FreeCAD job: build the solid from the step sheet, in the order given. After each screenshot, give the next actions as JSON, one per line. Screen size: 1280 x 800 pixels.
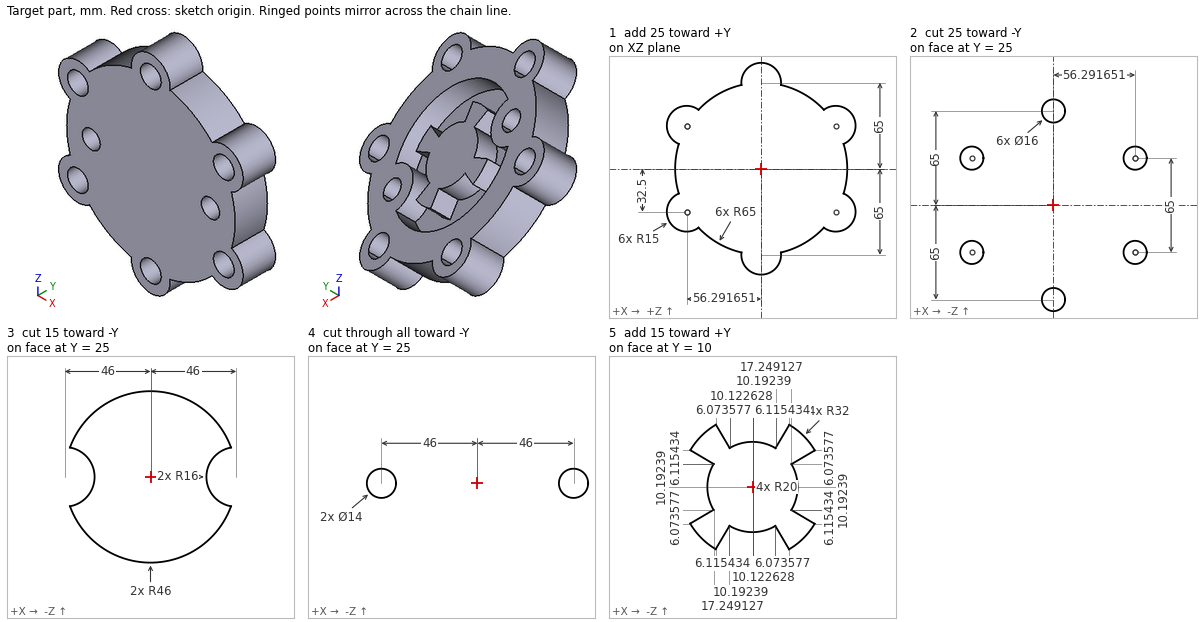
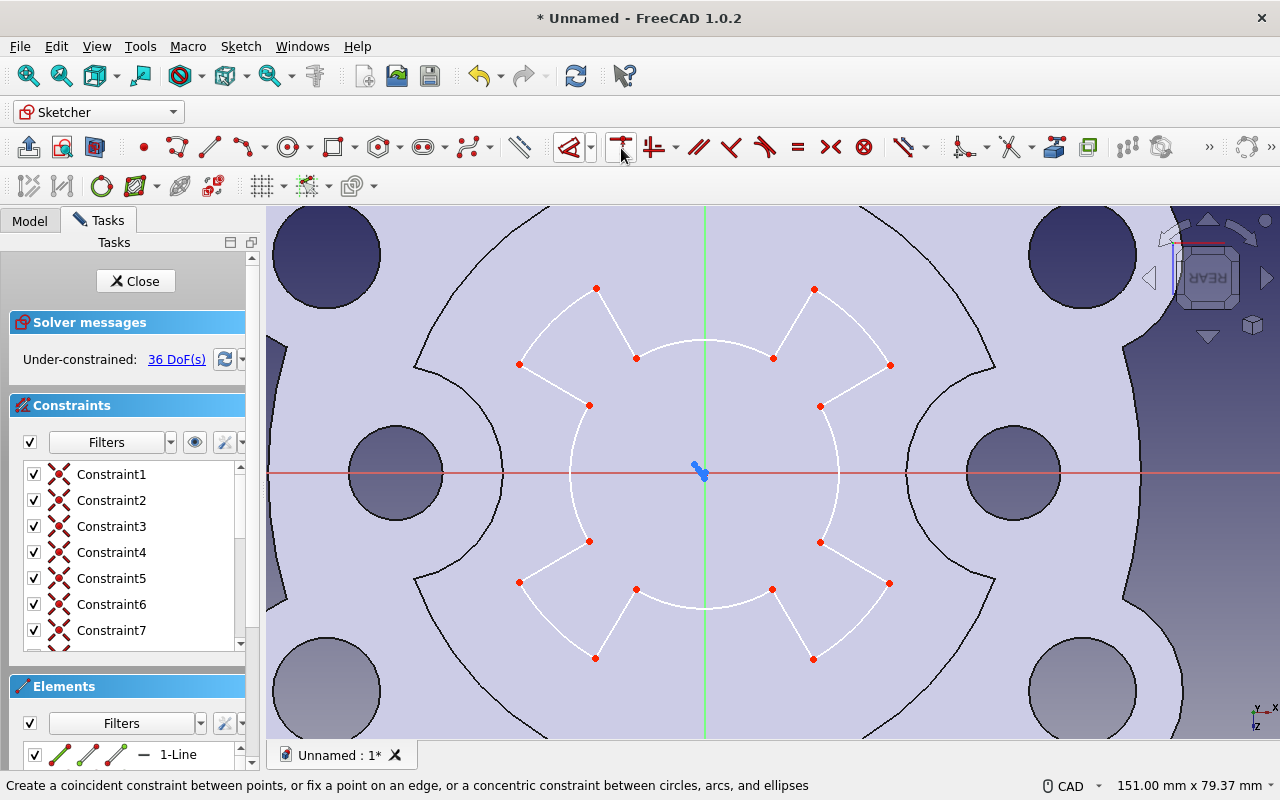
{"action": "left_click", "coordinate": [836, 503]}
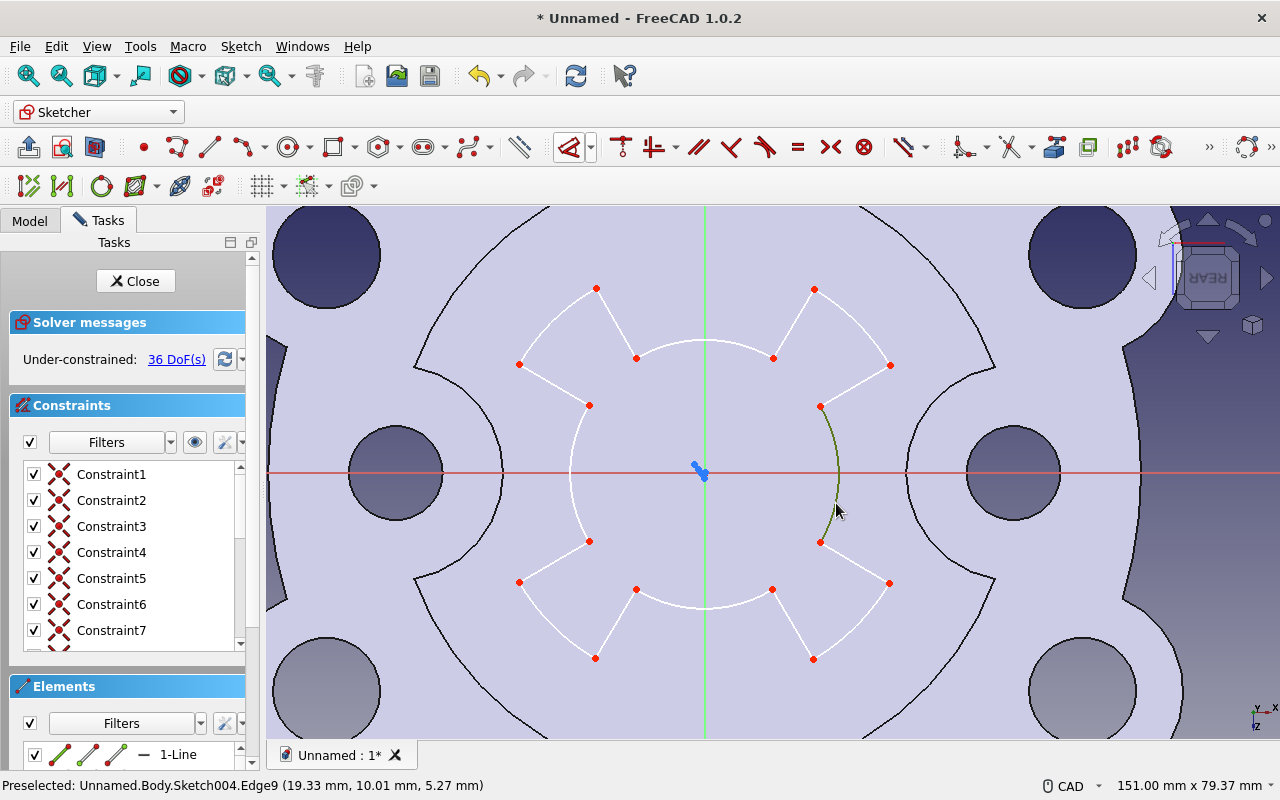
{"action": "left_click", "coordinate": [569, 307]}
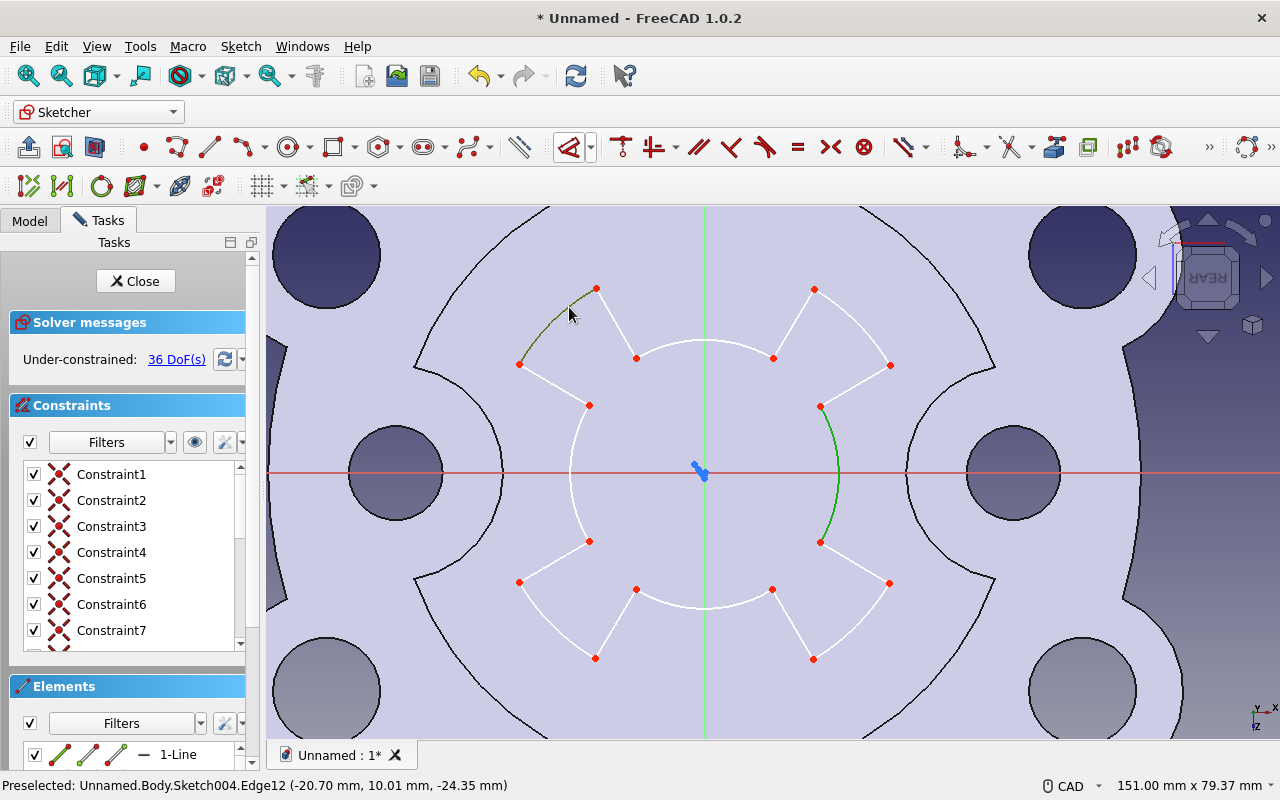
{"action": "left_click", "coordinate": [621, 148]}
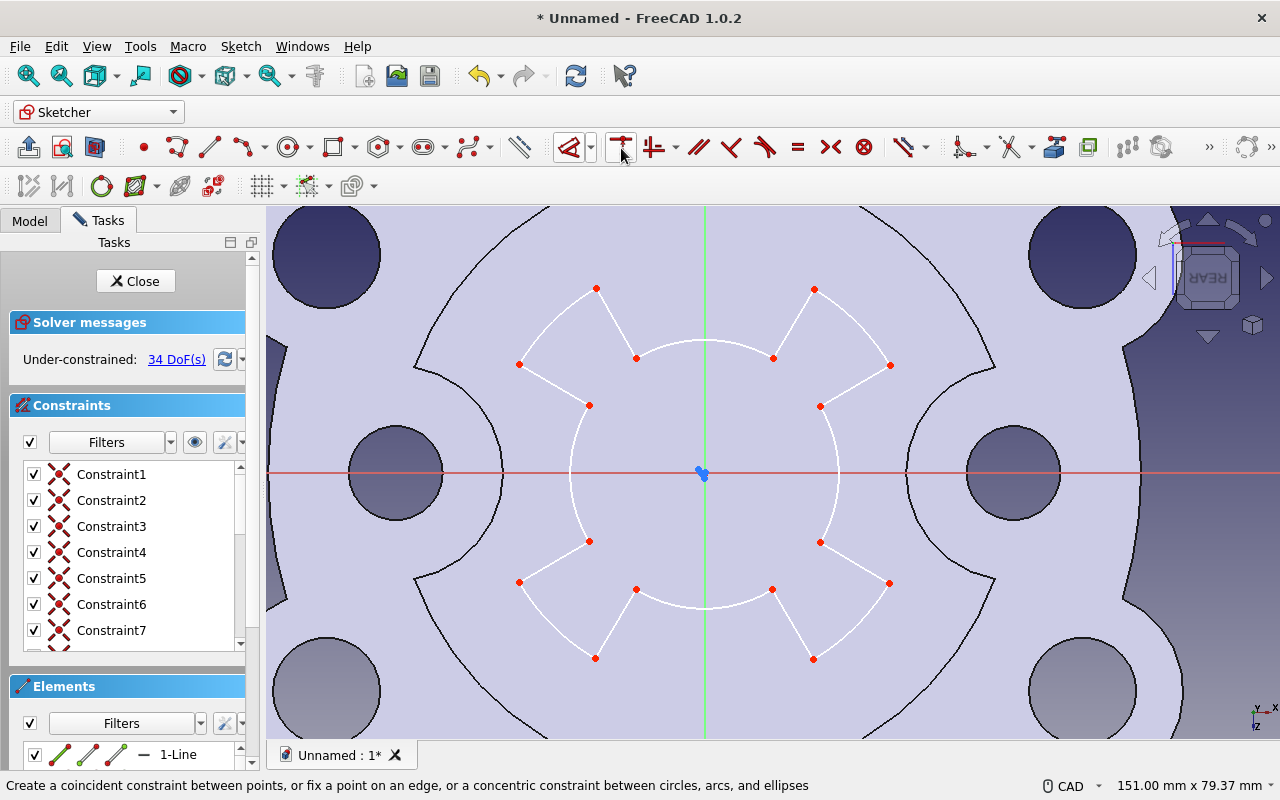
{"action": "left_click", "coordinate": [836, 503]}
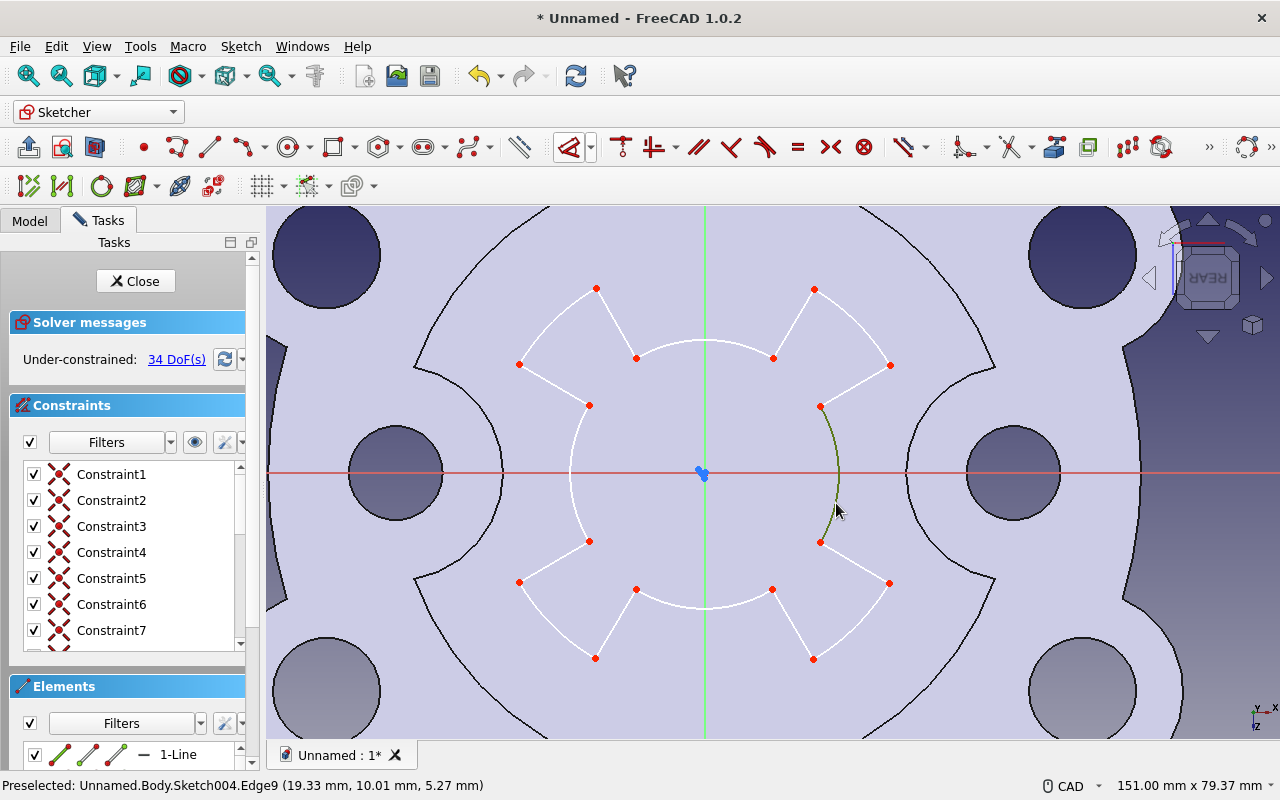
{"action": "left_click", "coordinate": [573, 445]}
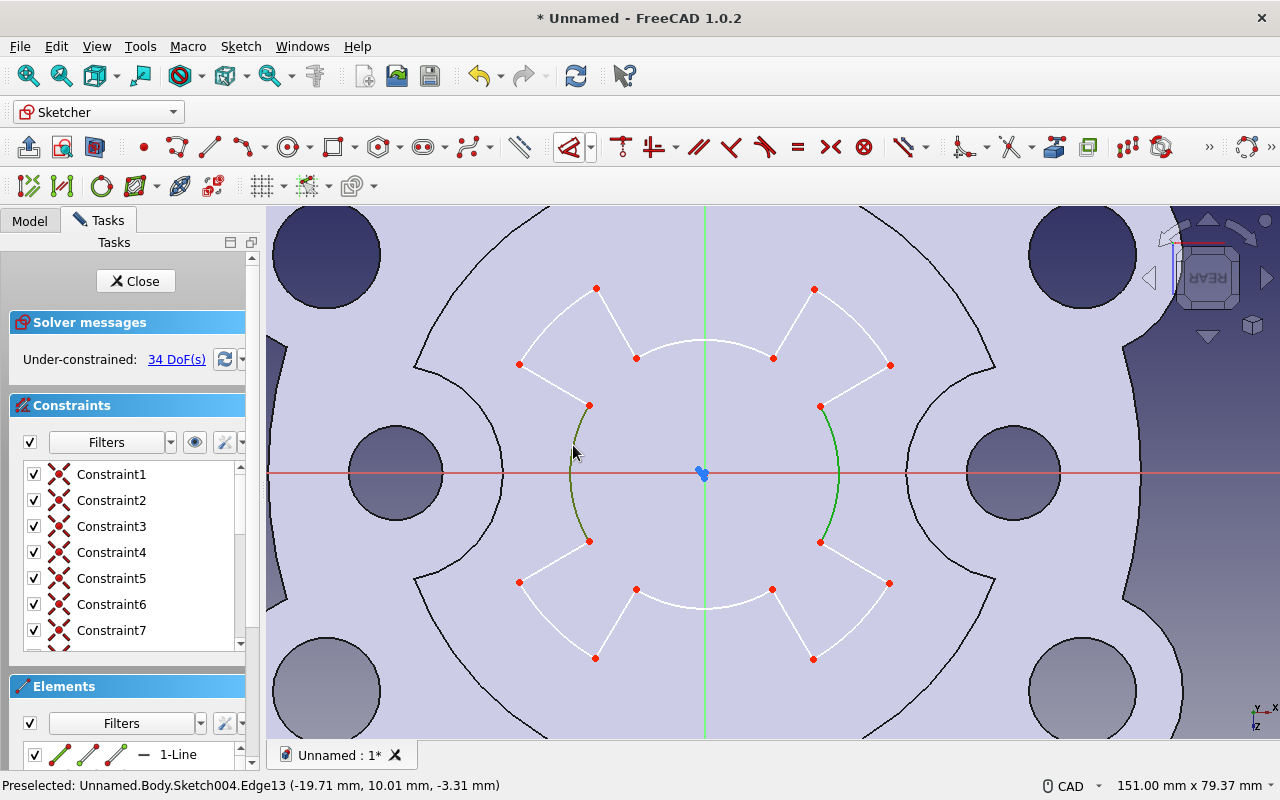
{"action": "left_click", "coordinate": [621, 148]}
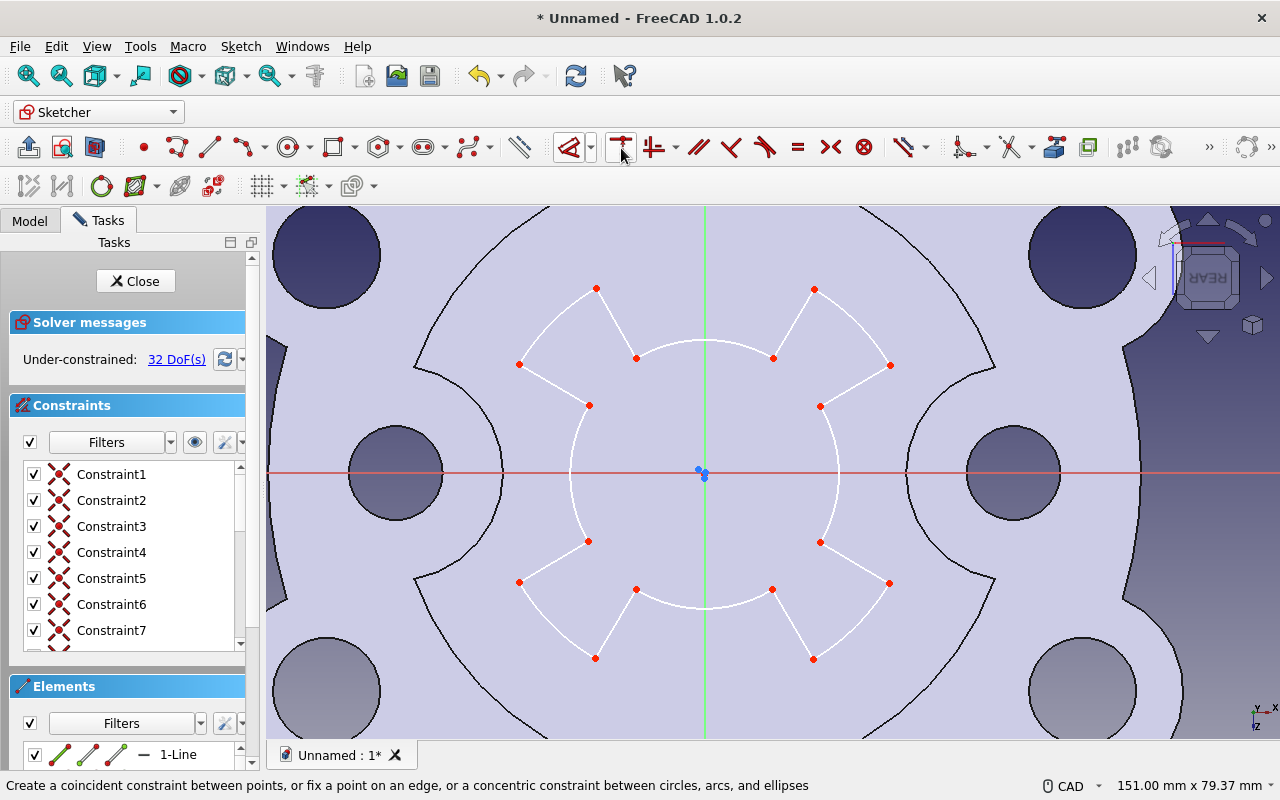
{"action": "left_click", "coordinate": [836, 503]}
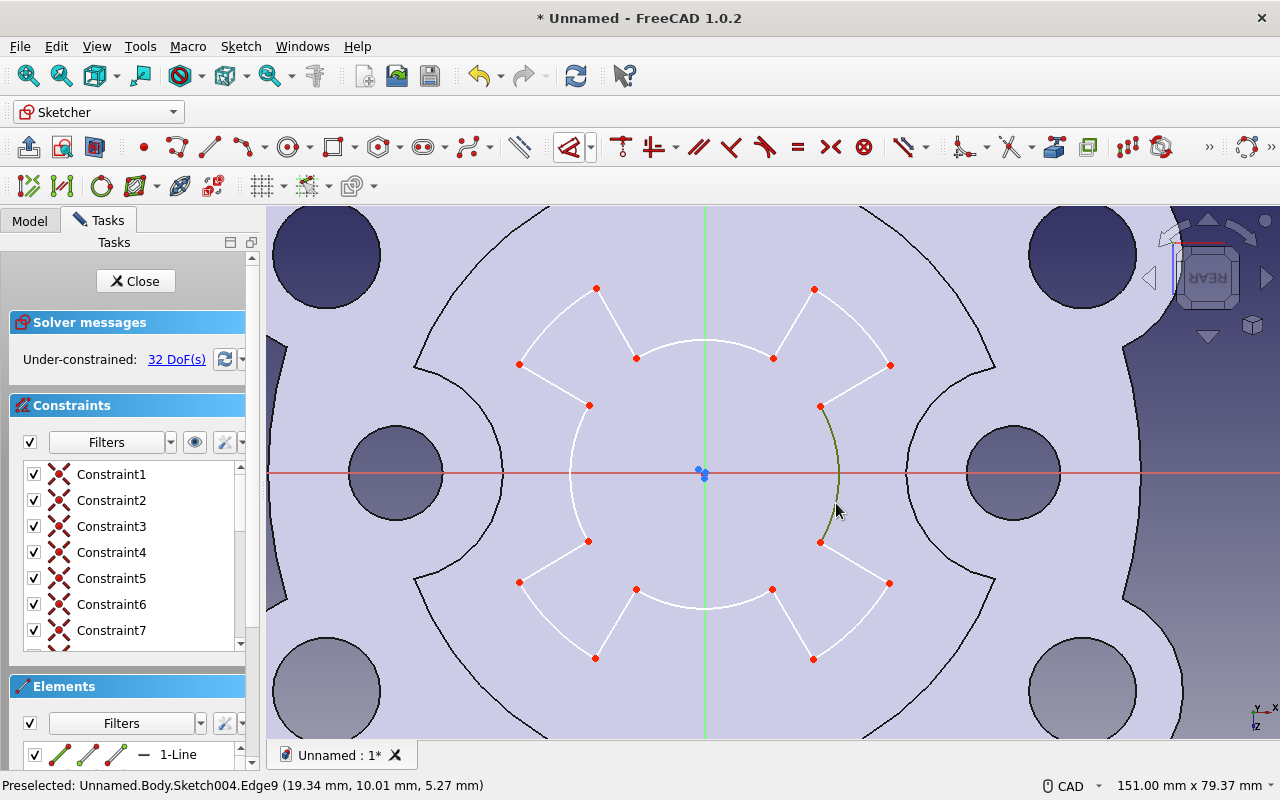
{"action": "left_click", "coordinate": [538, 609]}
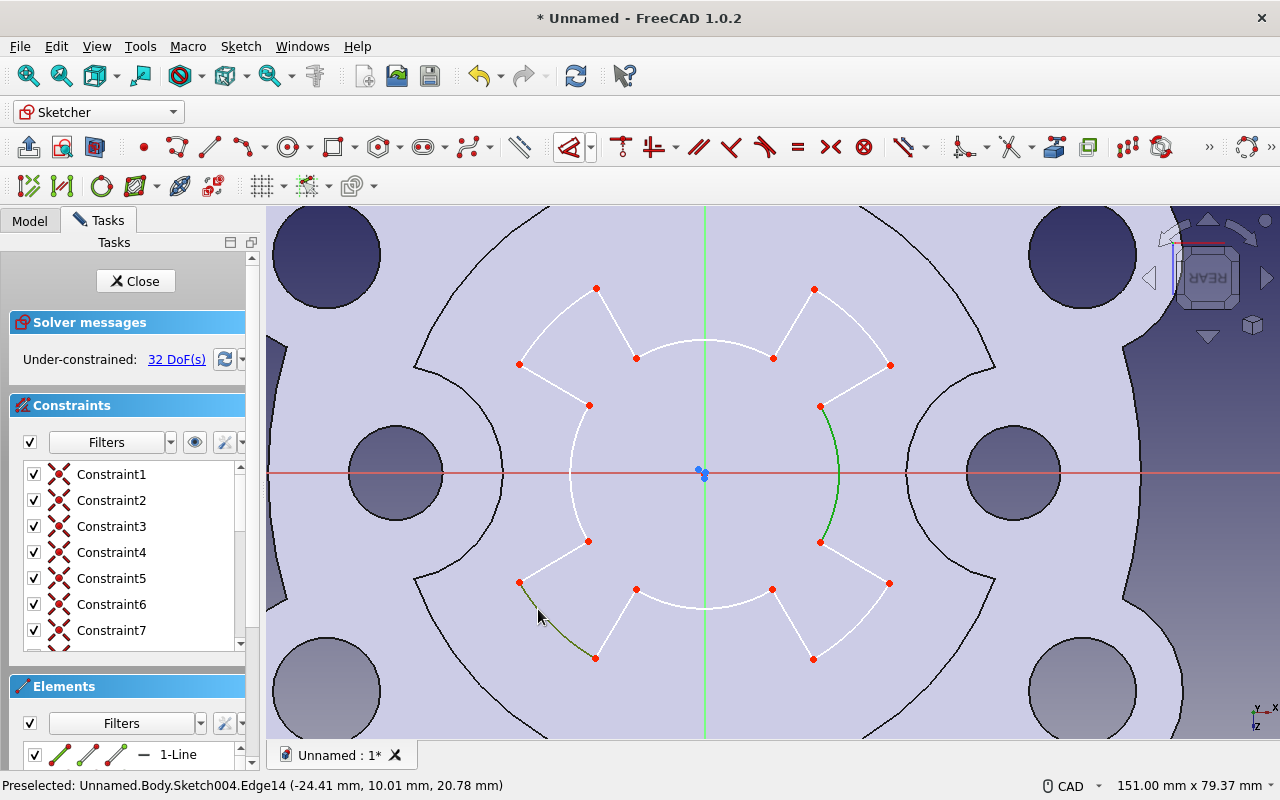
{"action": "left_click", "coordinate": [621, 148]}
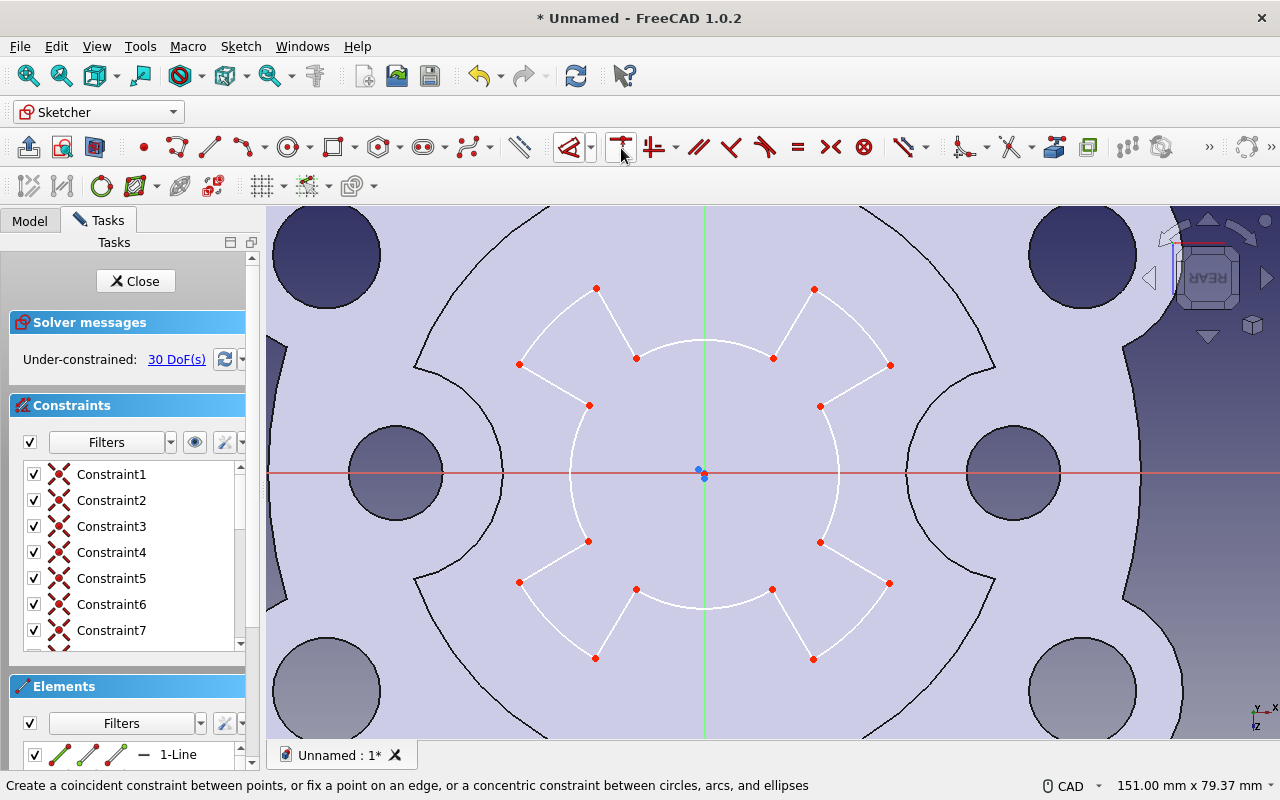
{"action": "left_click", "coordinate": [836, 503]}